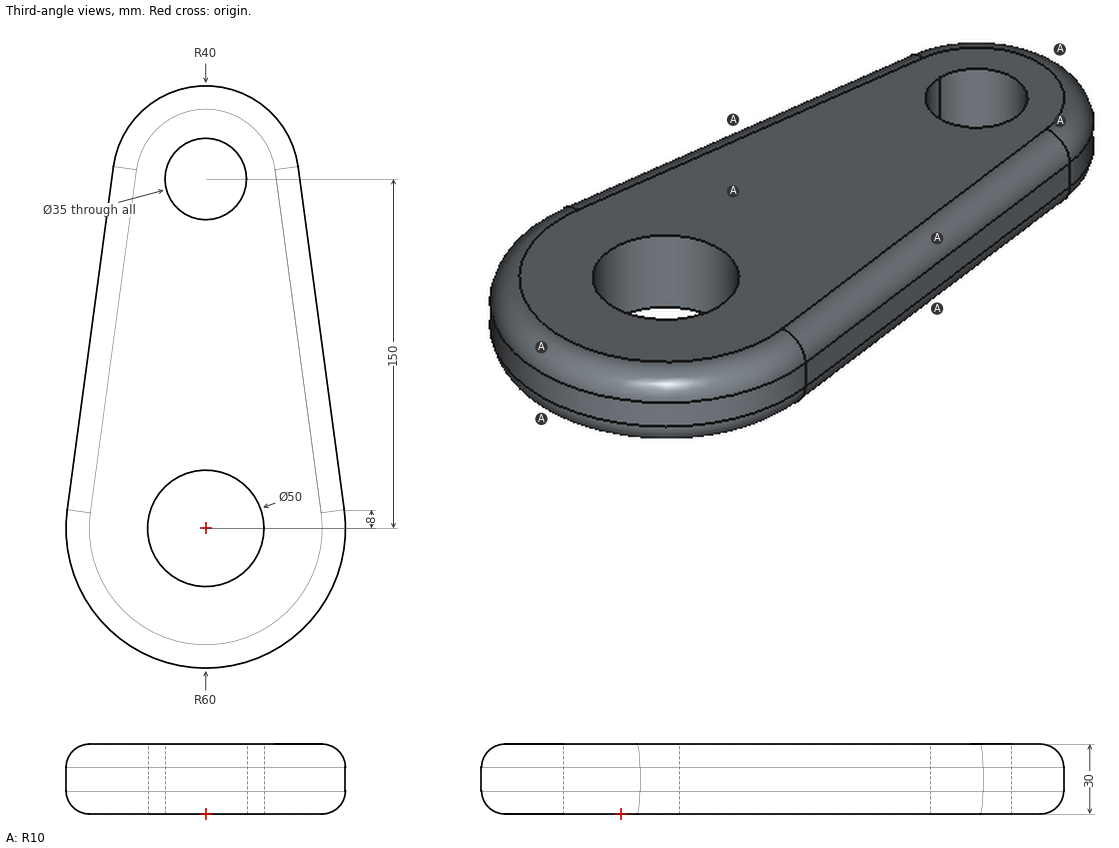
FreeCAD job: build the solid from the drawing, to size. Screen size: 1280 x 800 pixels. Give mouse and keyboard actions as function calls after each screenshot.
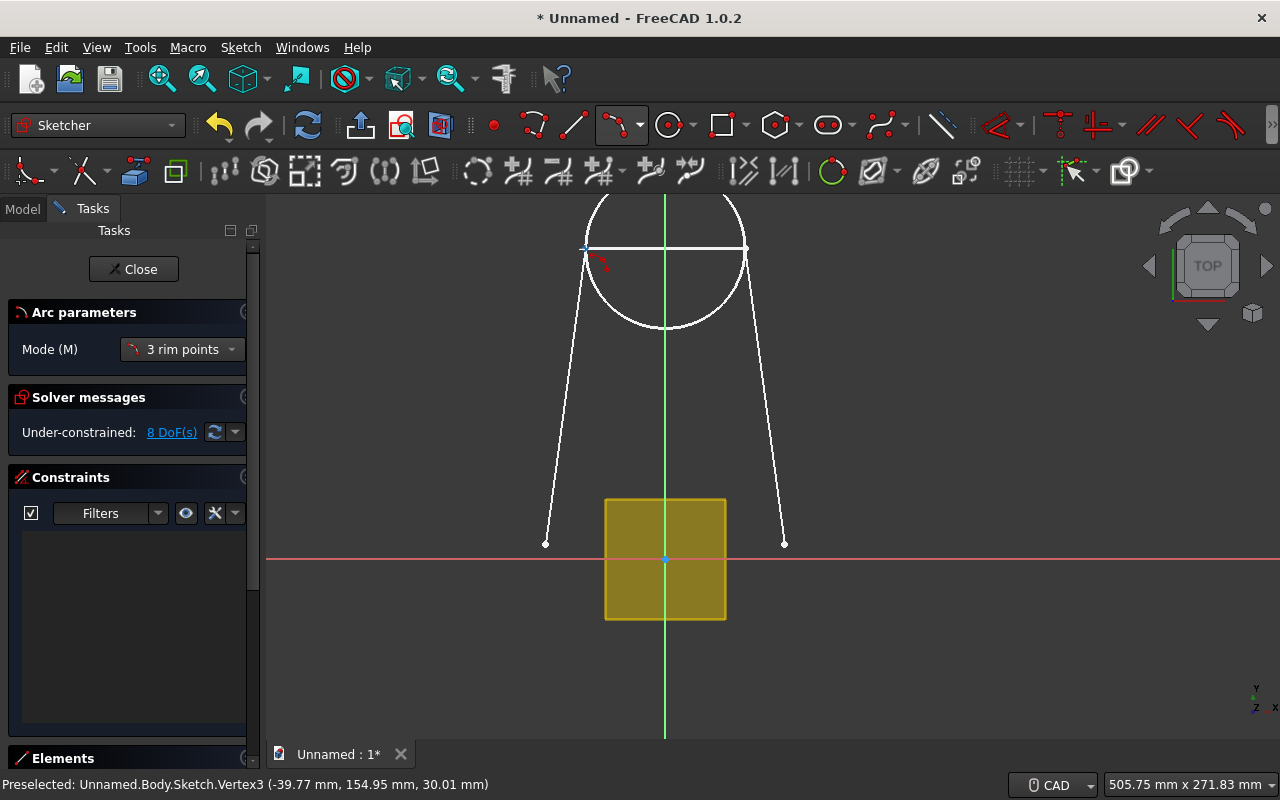
scroll(784, 542, down, 2)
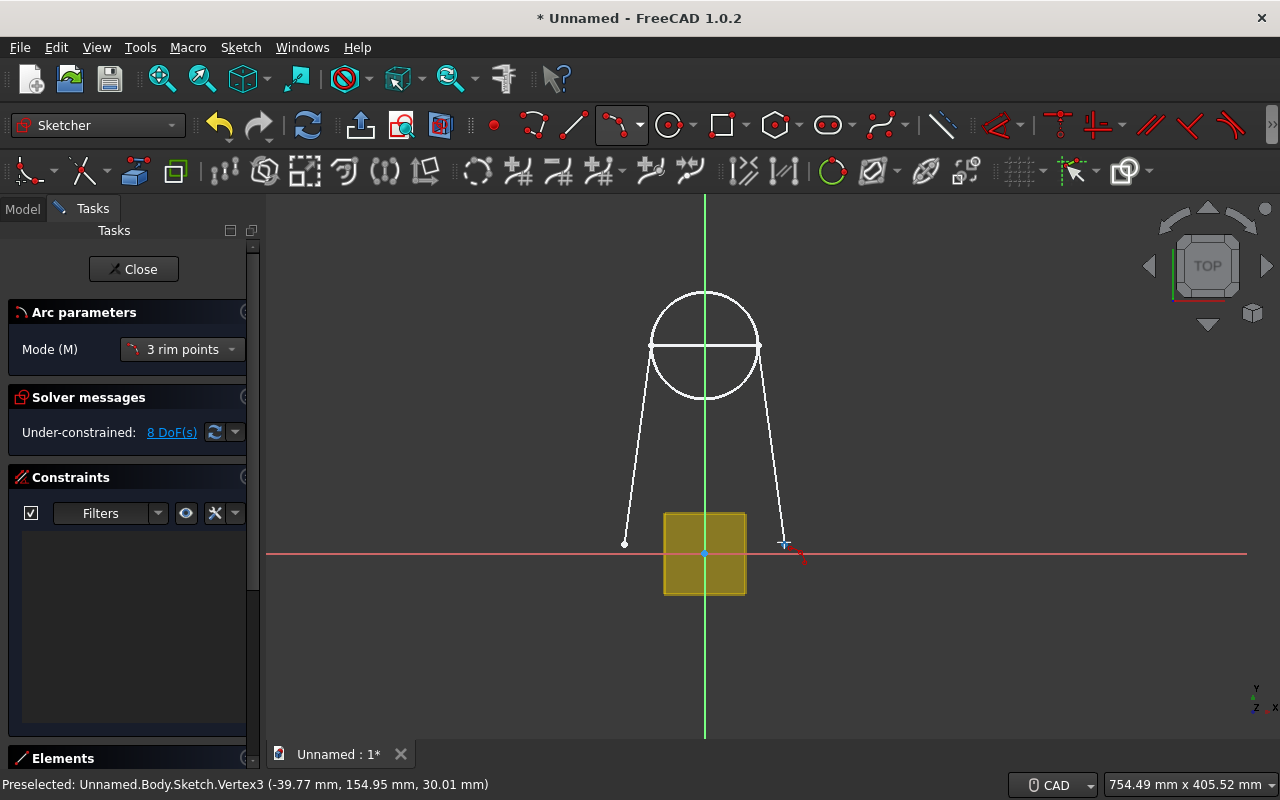
click(720, 301)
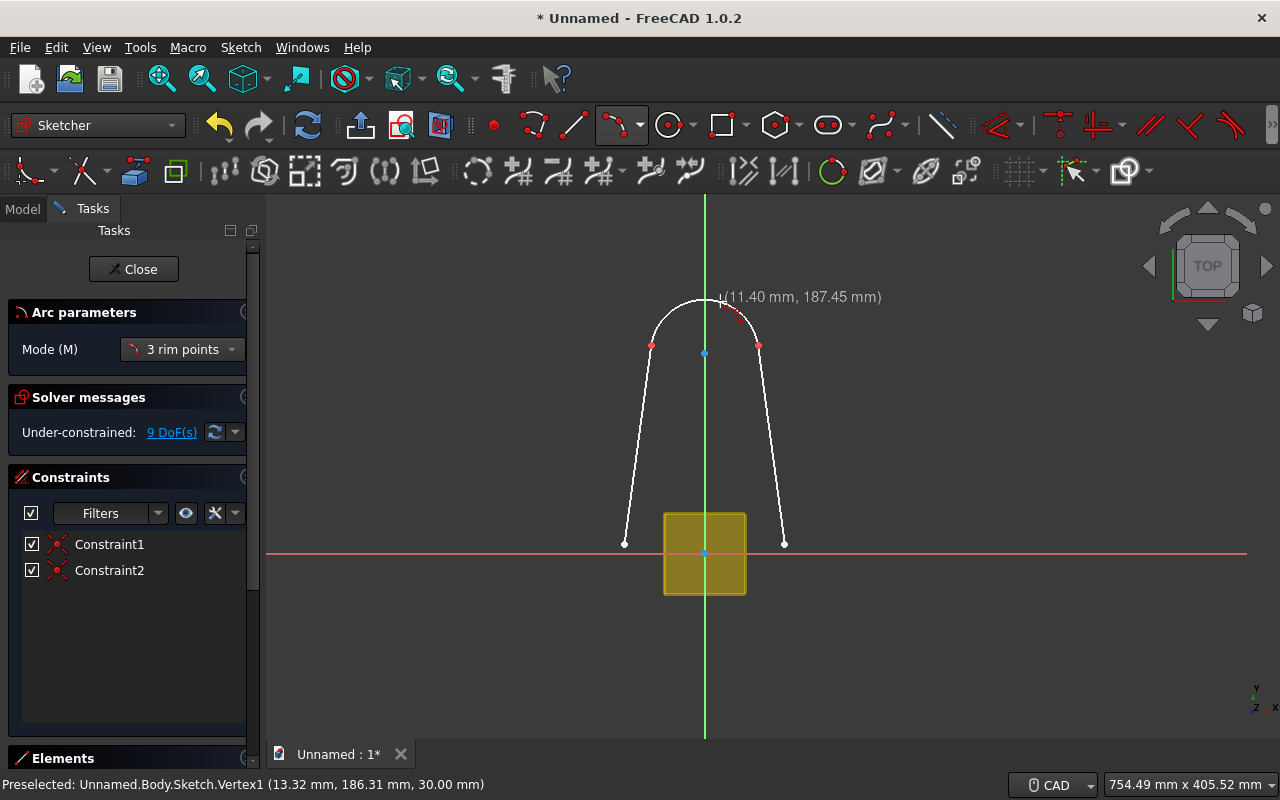
scroll(625, 543, up, 2)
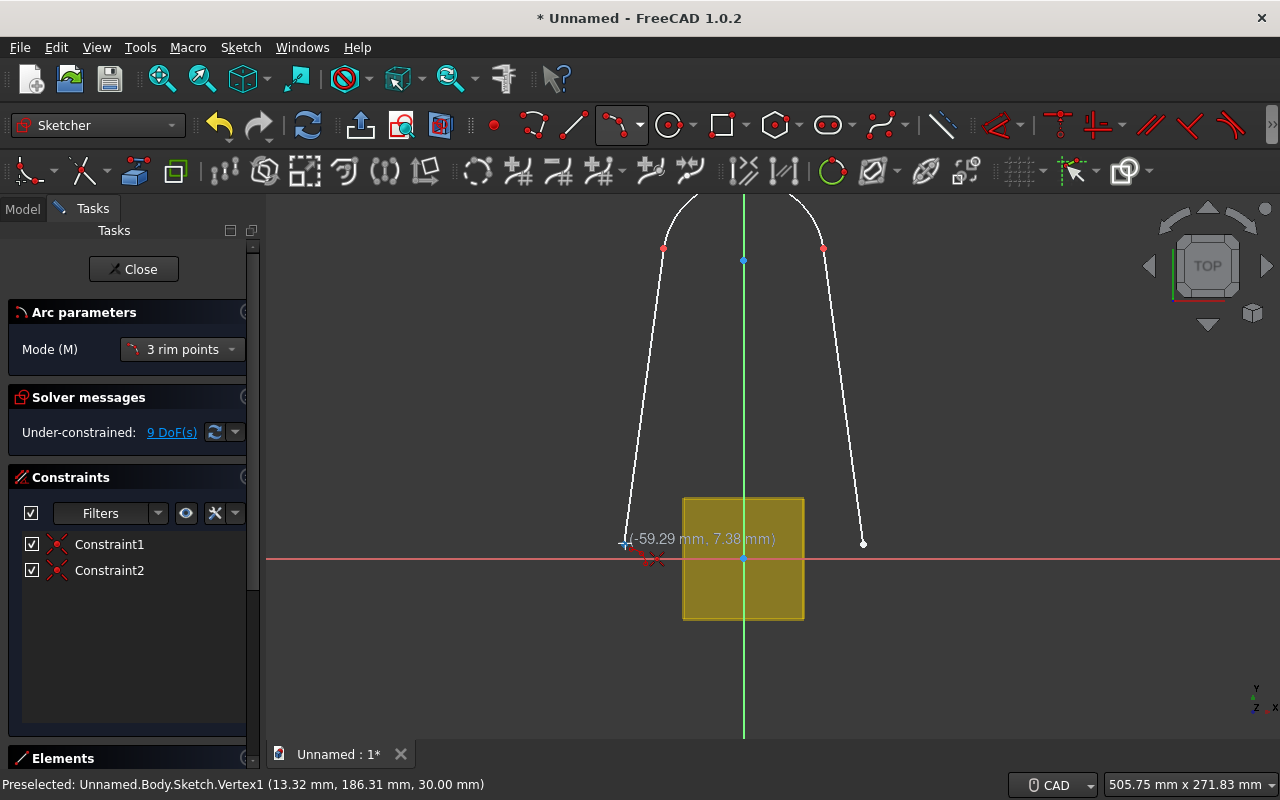
click(624, 544)
click(863, 544)
click(703, 672)
key(Escape)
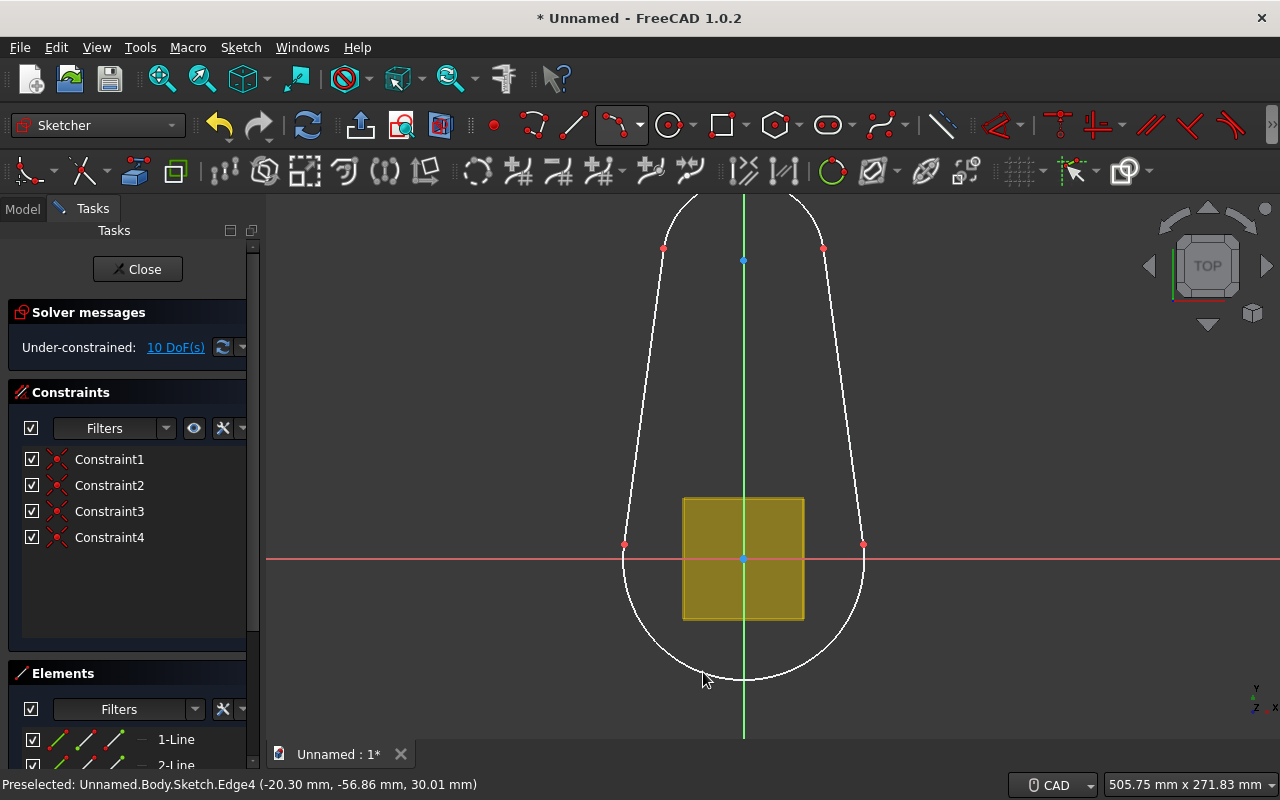
click(851, 455)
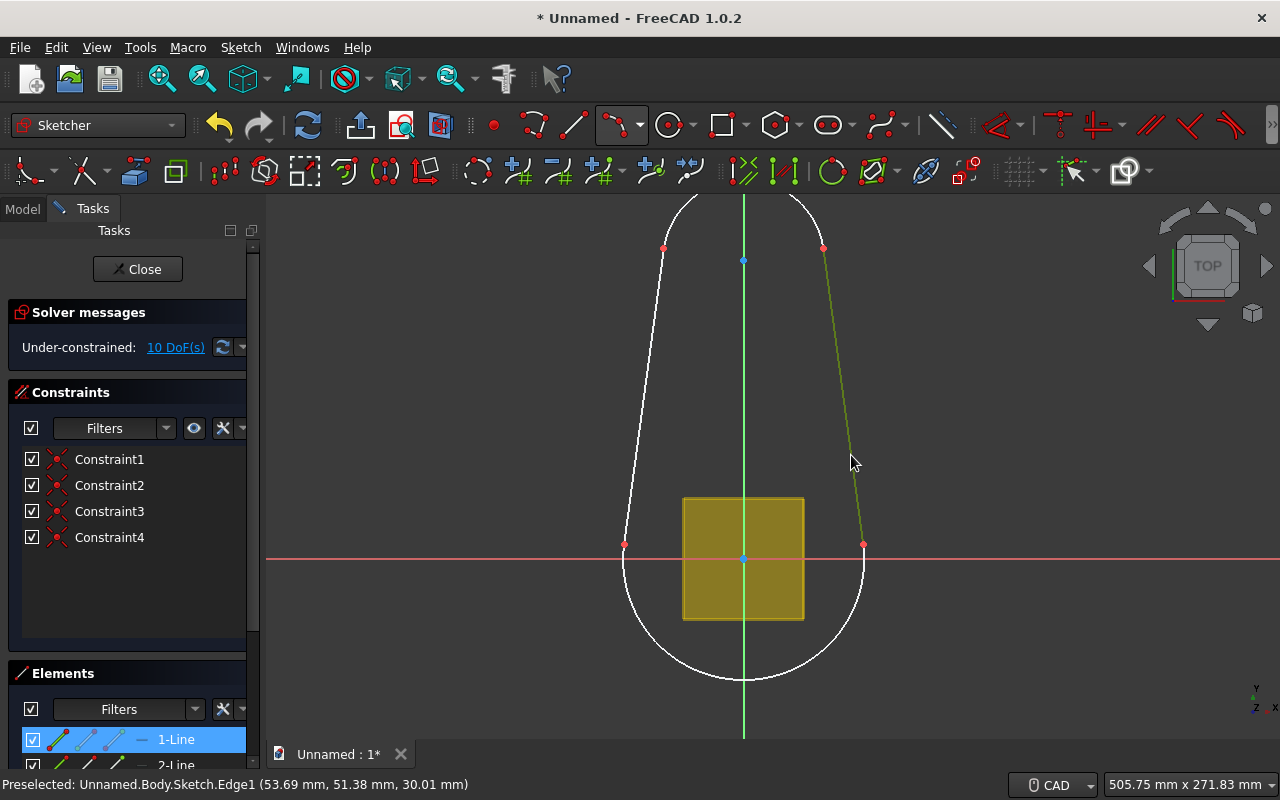
scroll(625, 543, down, 2)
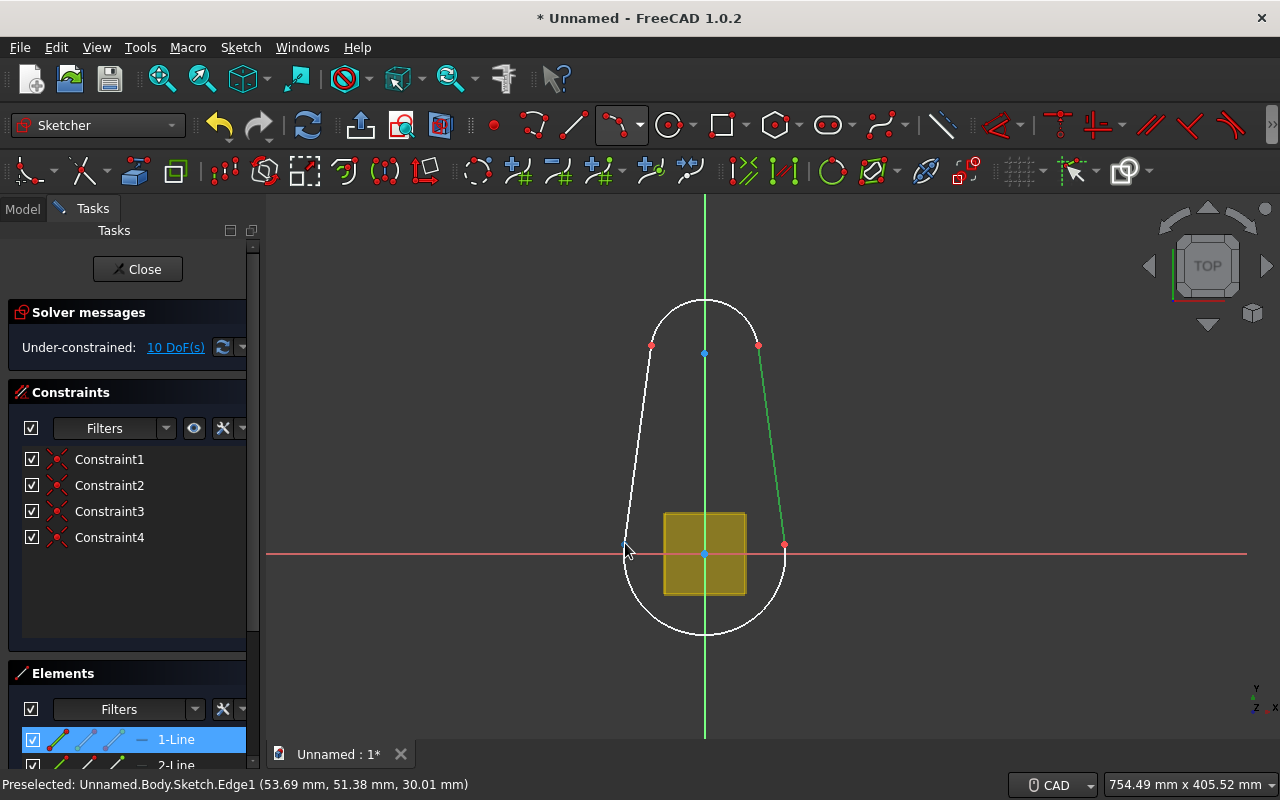
click(734, 308)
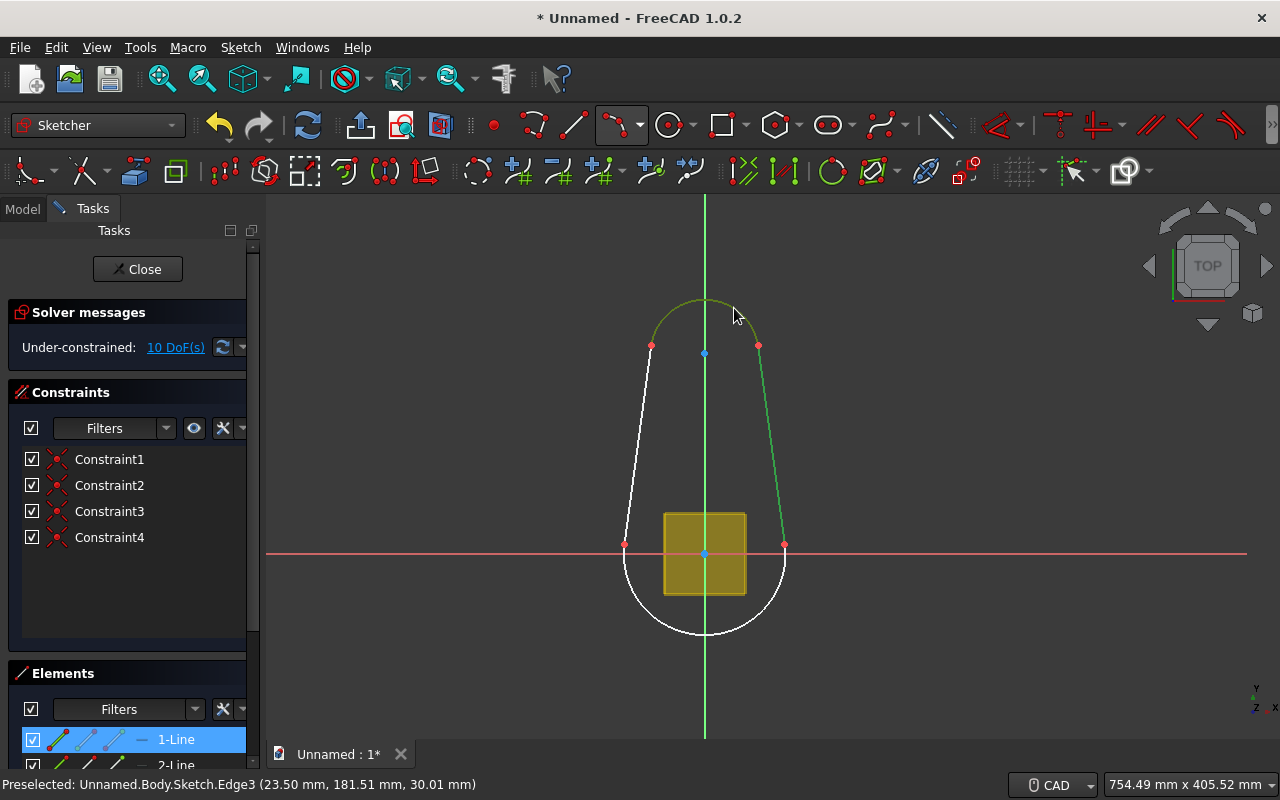
click(1232, 126)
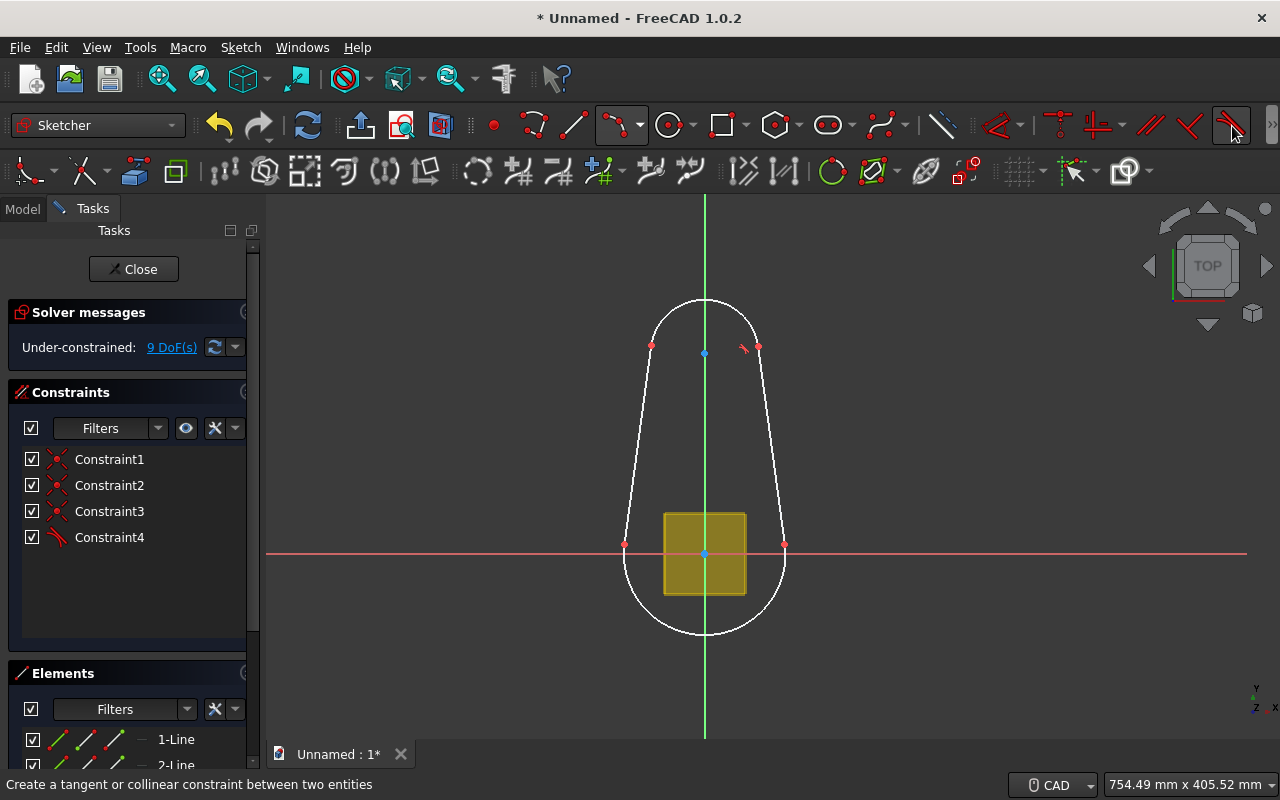
click(643, 405)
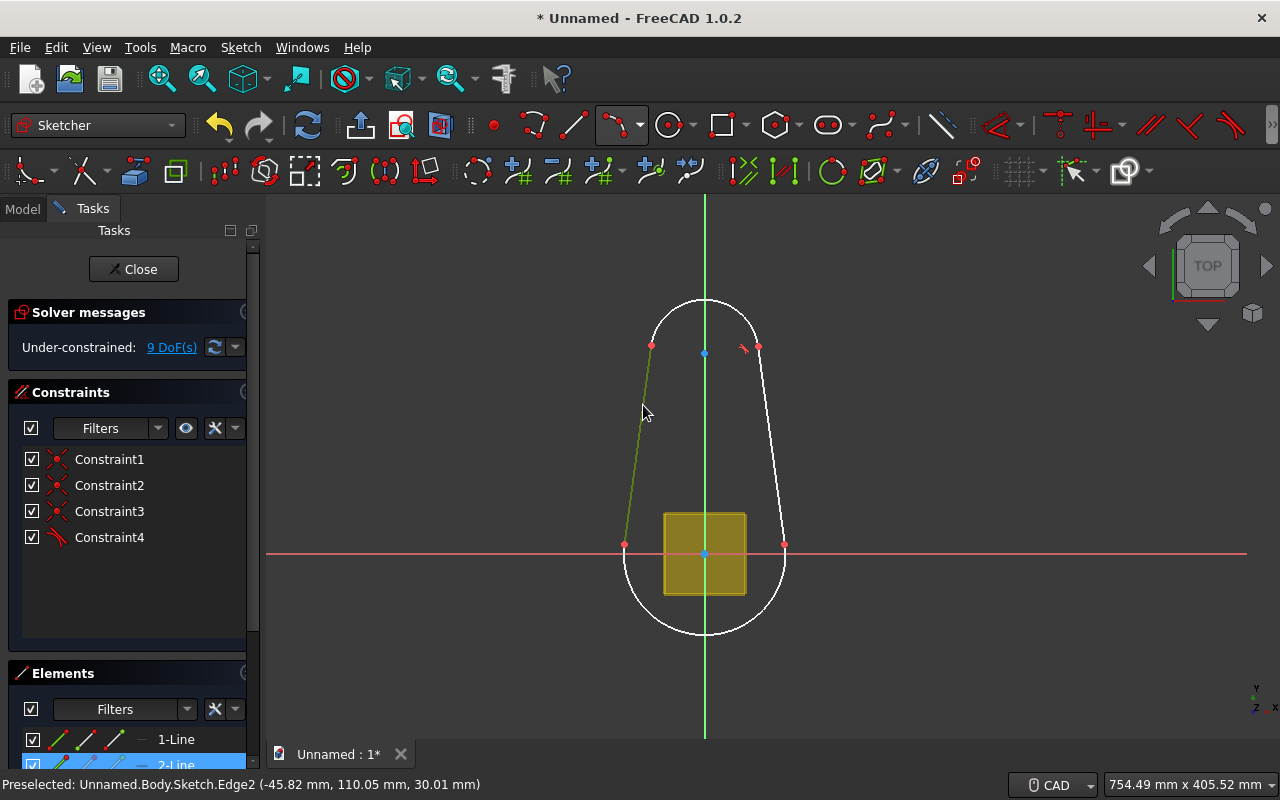
click(734, 309)